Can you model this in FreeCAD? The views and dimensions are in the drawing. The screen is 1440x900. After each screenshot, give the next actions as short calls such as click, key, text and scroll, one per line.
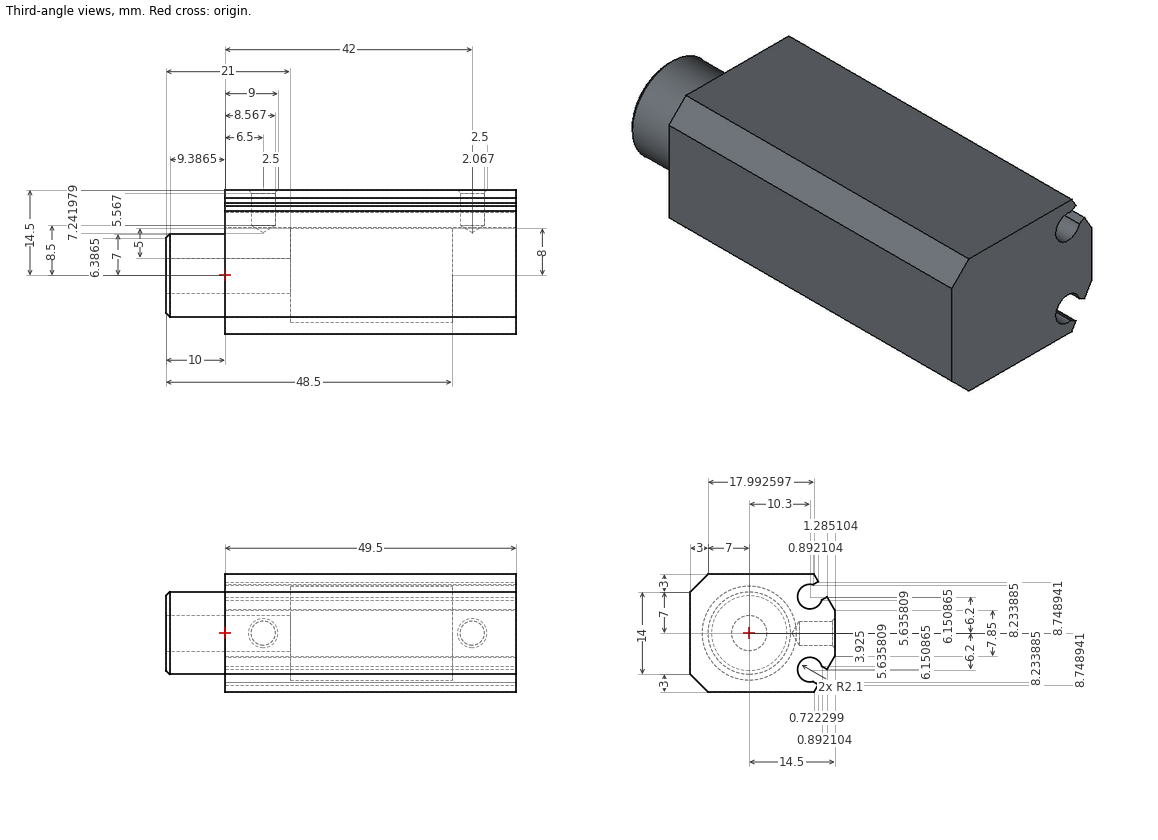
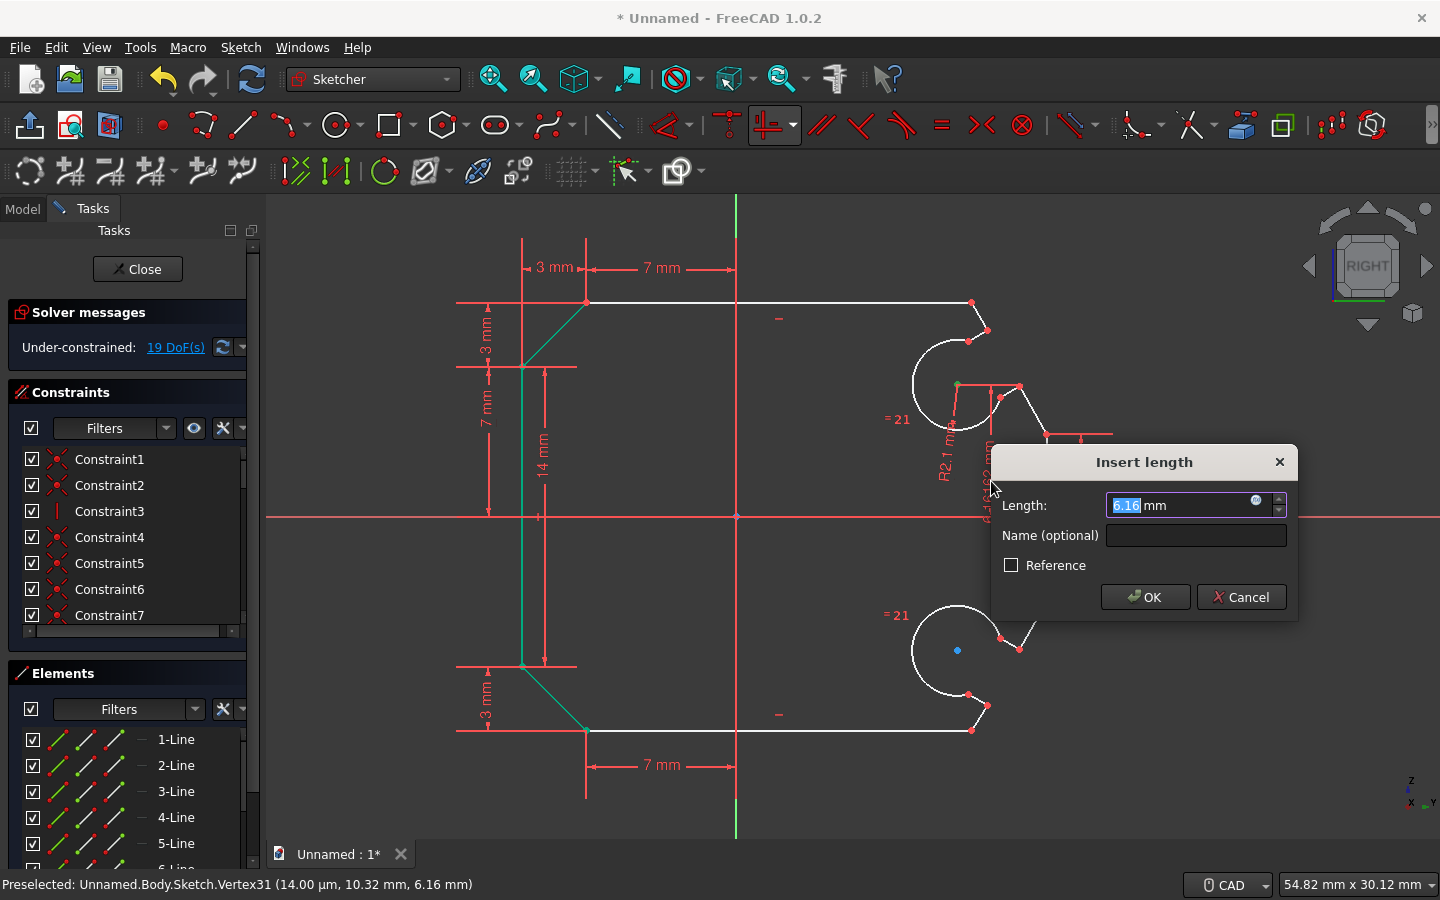
text(6.2)
key(Return)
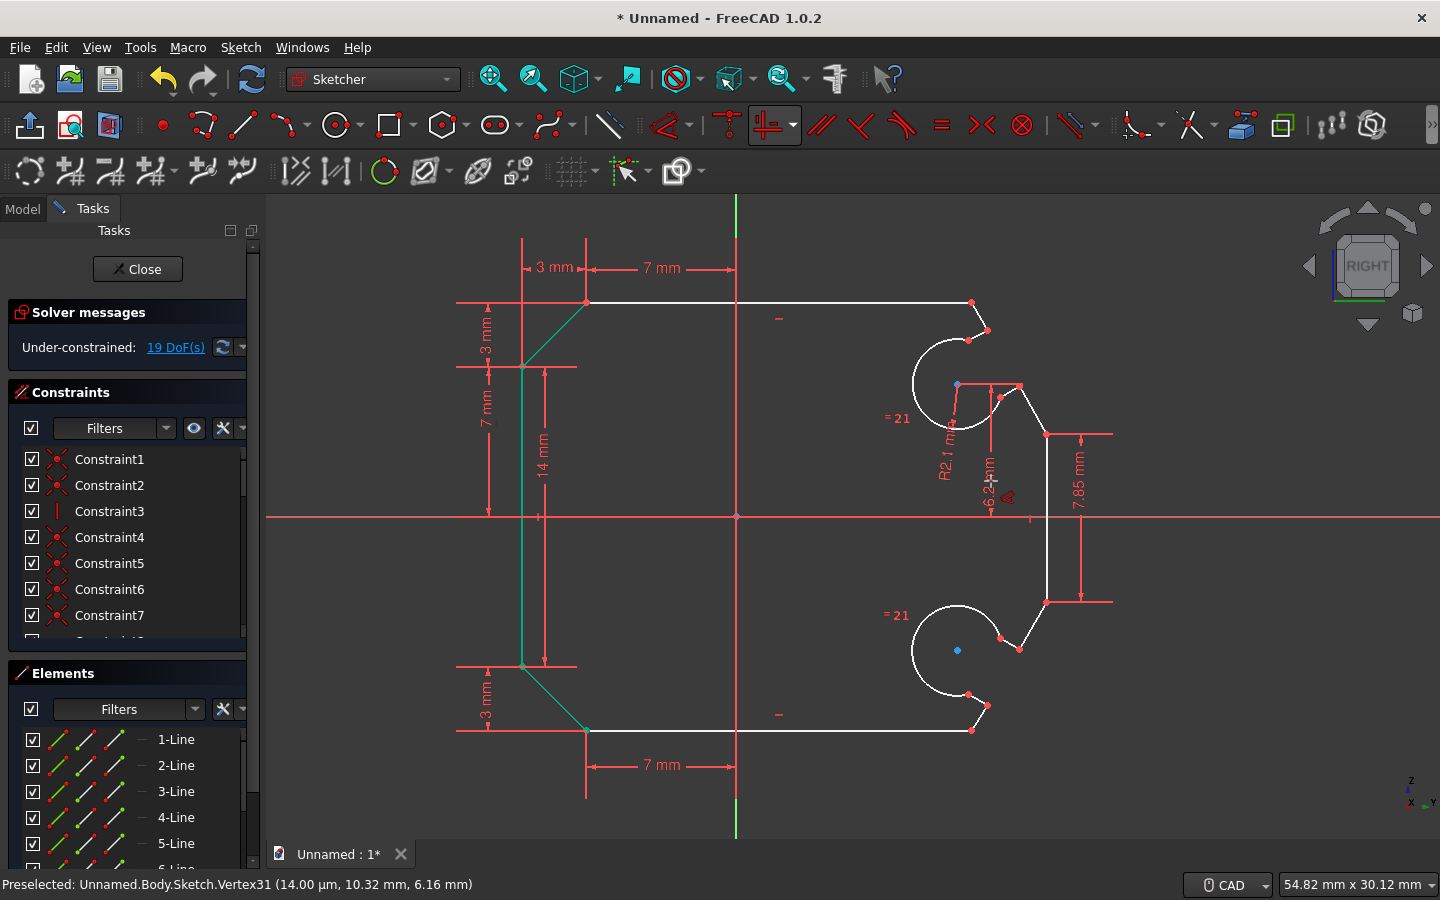
click(957, 651)
click(991, 584)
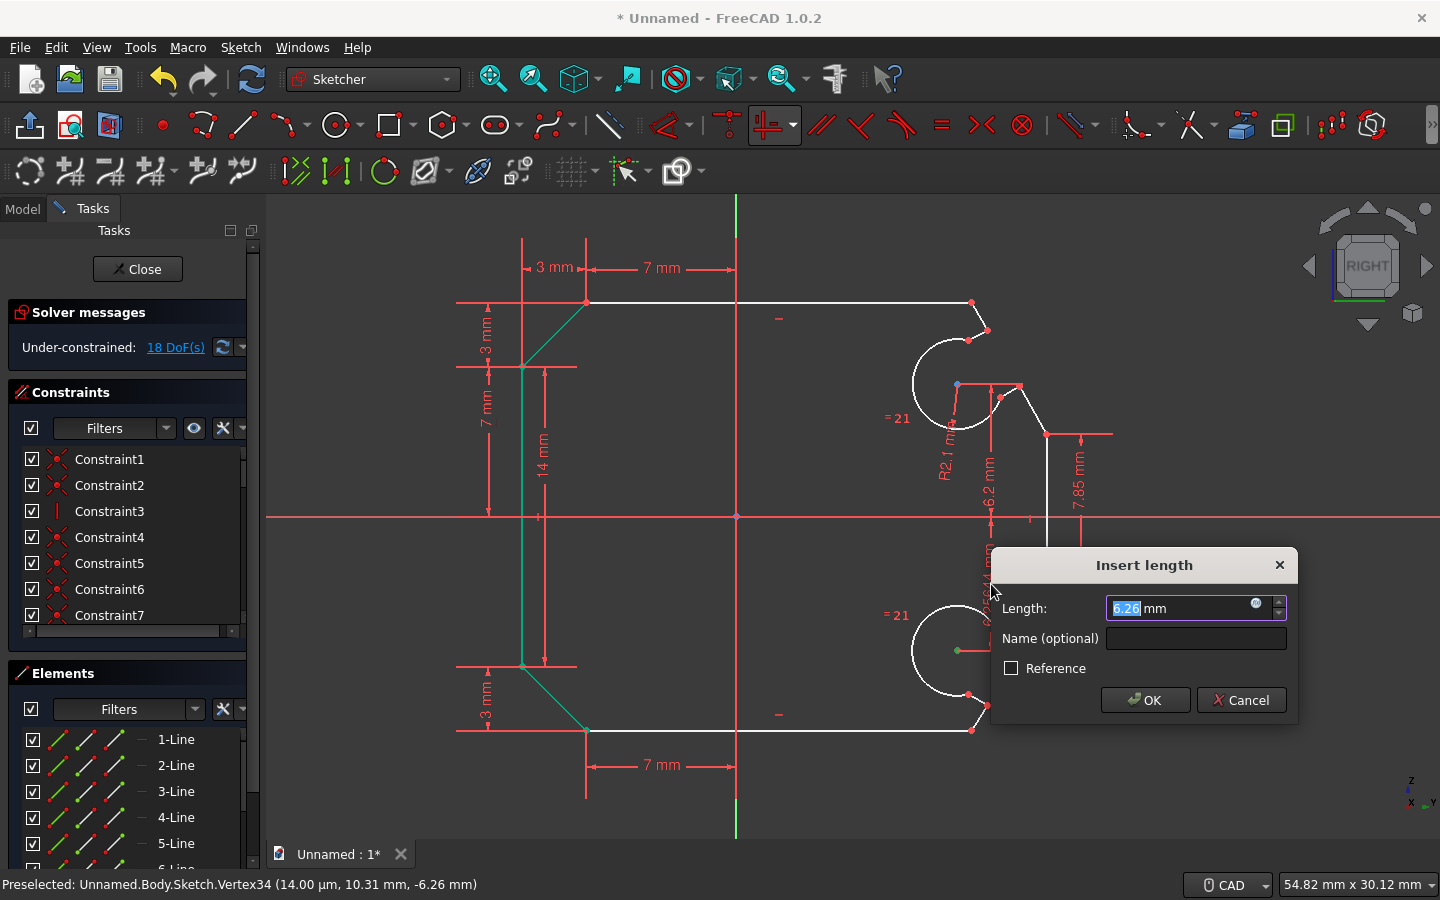
text(6.2)
key(Return)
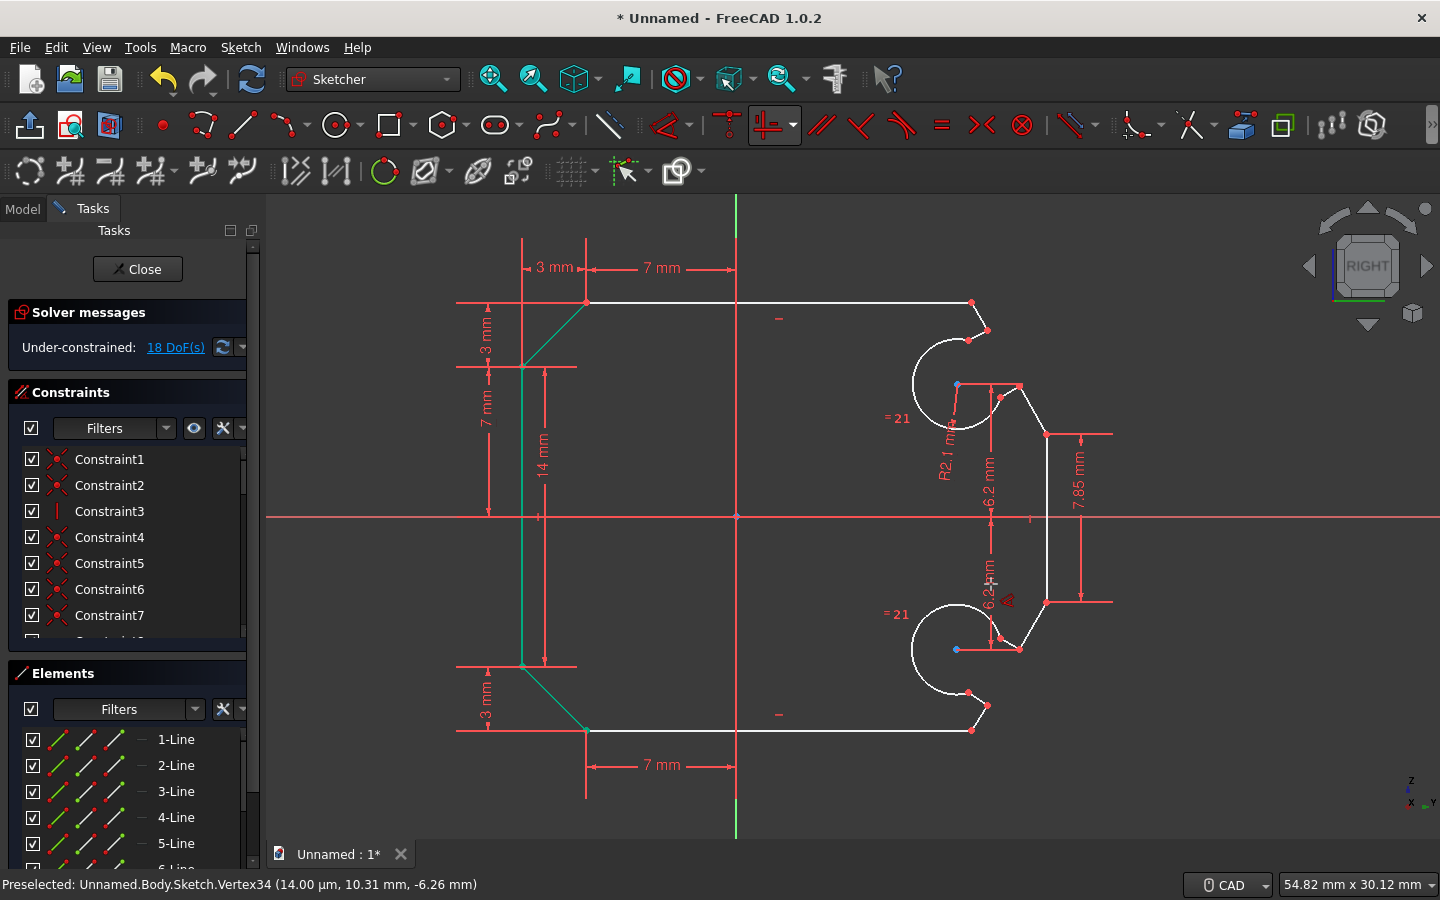
click(1047, 602)
click(892, 636)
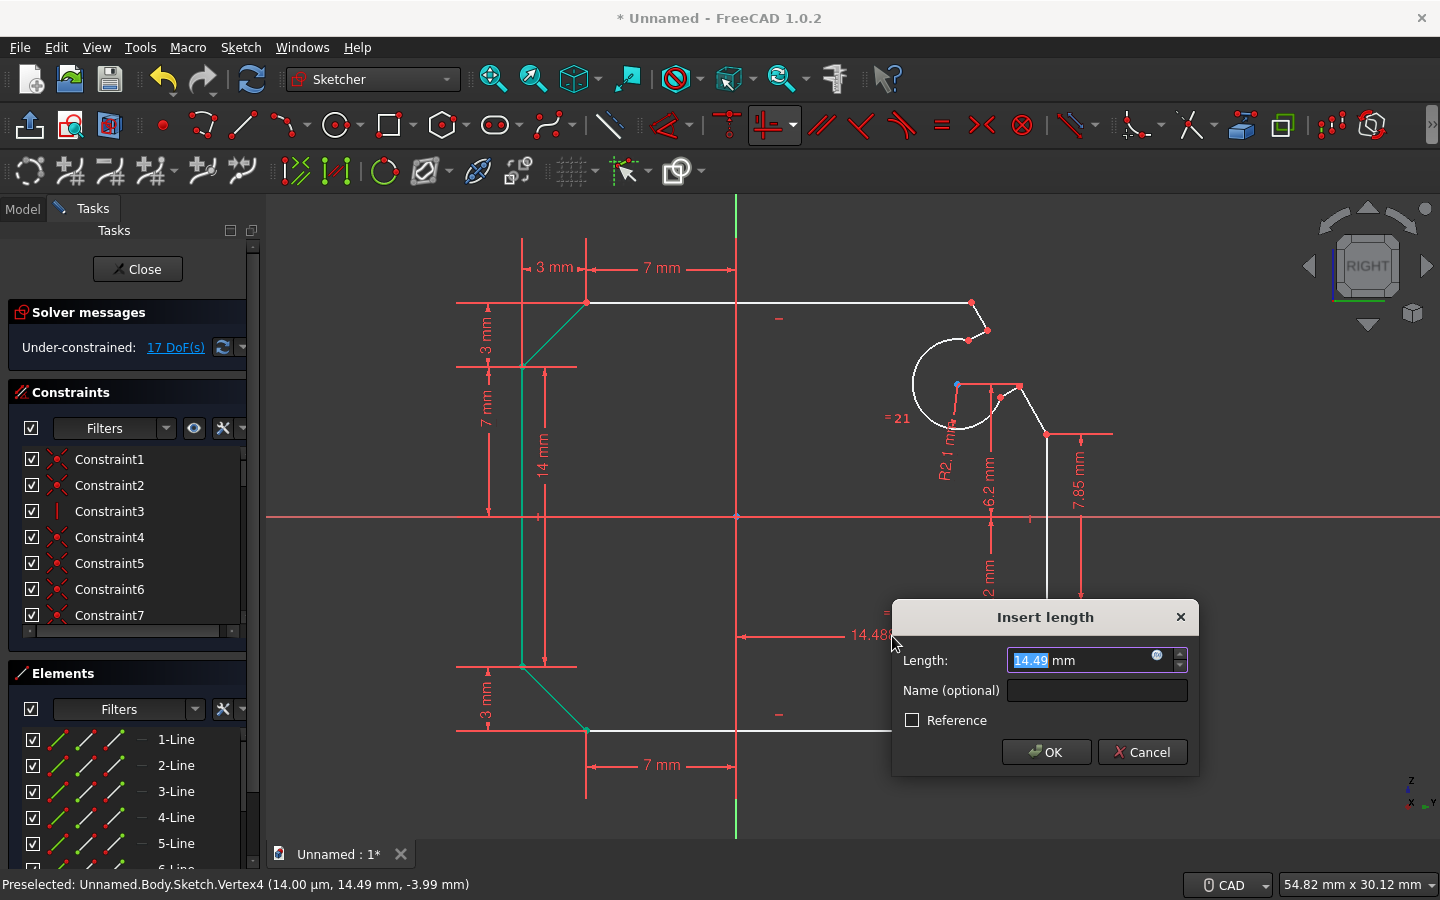
text(14.5)
key(Return)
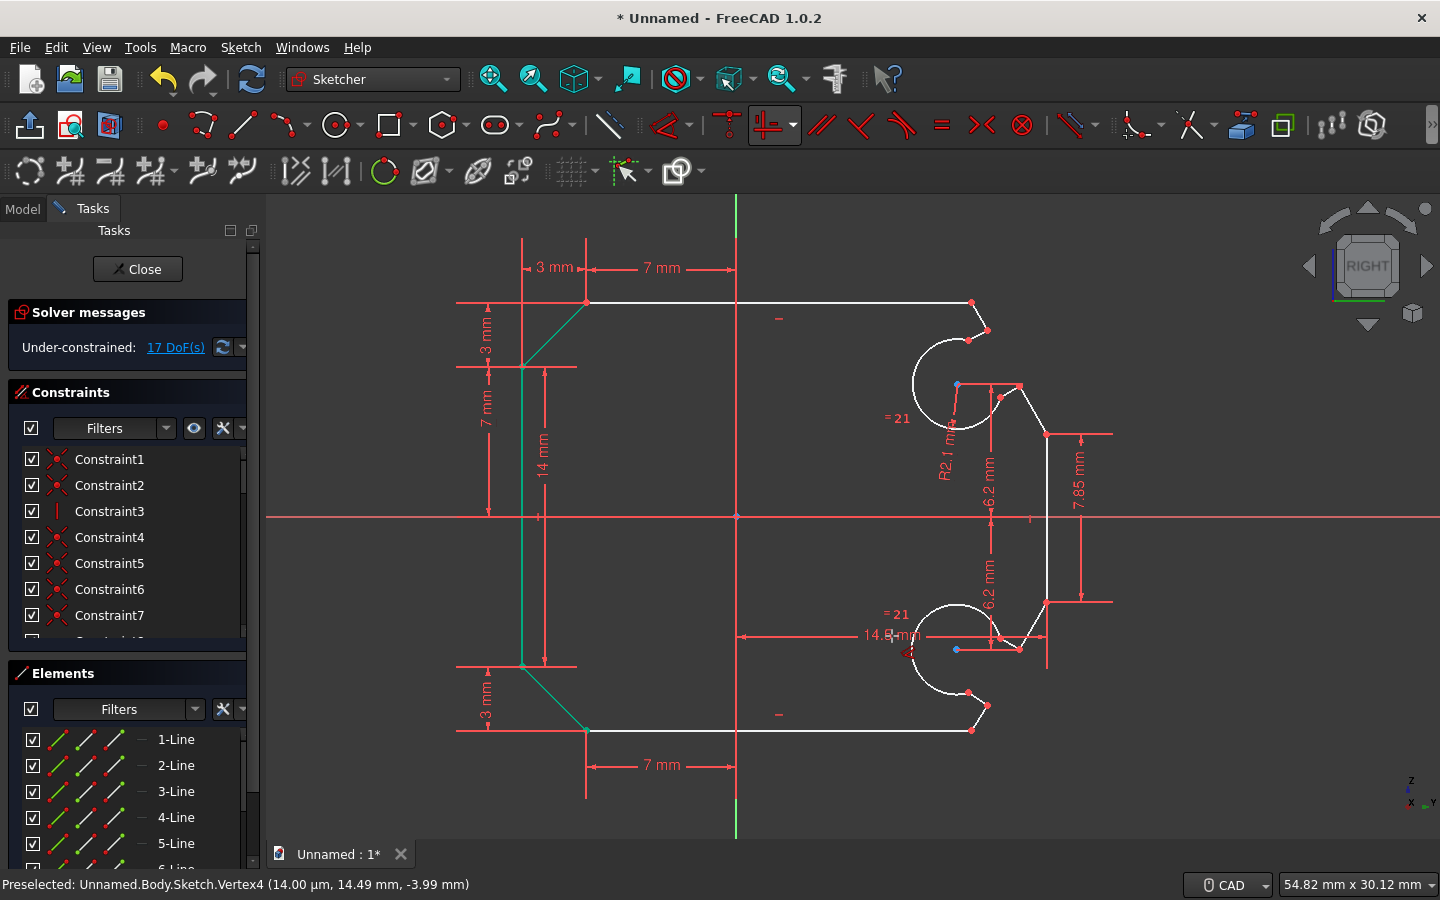
click(958, 384)
click(847, 350)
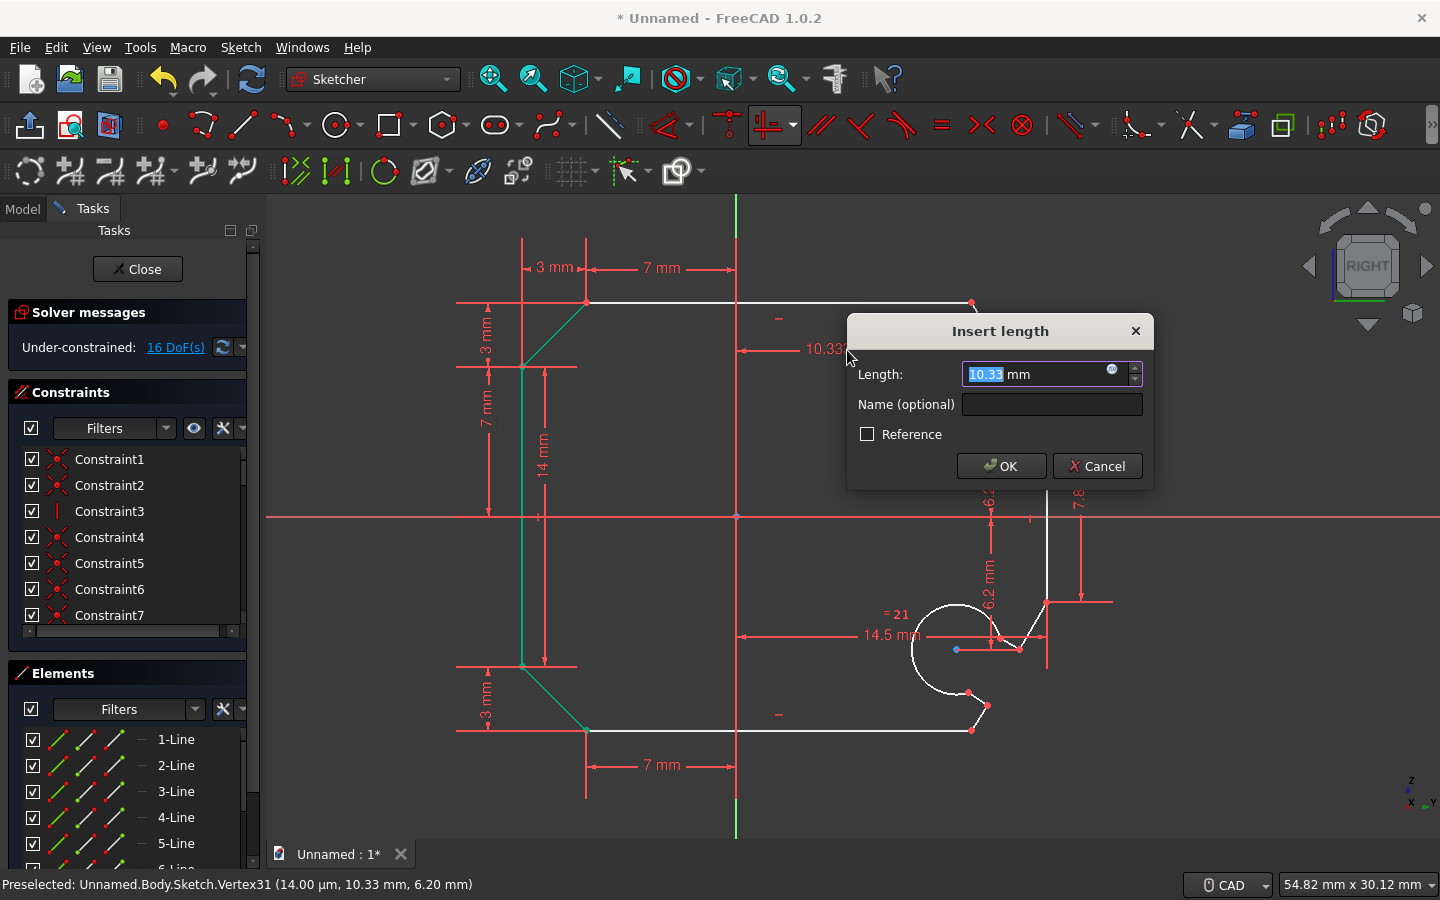
text(10.3)
key(Return)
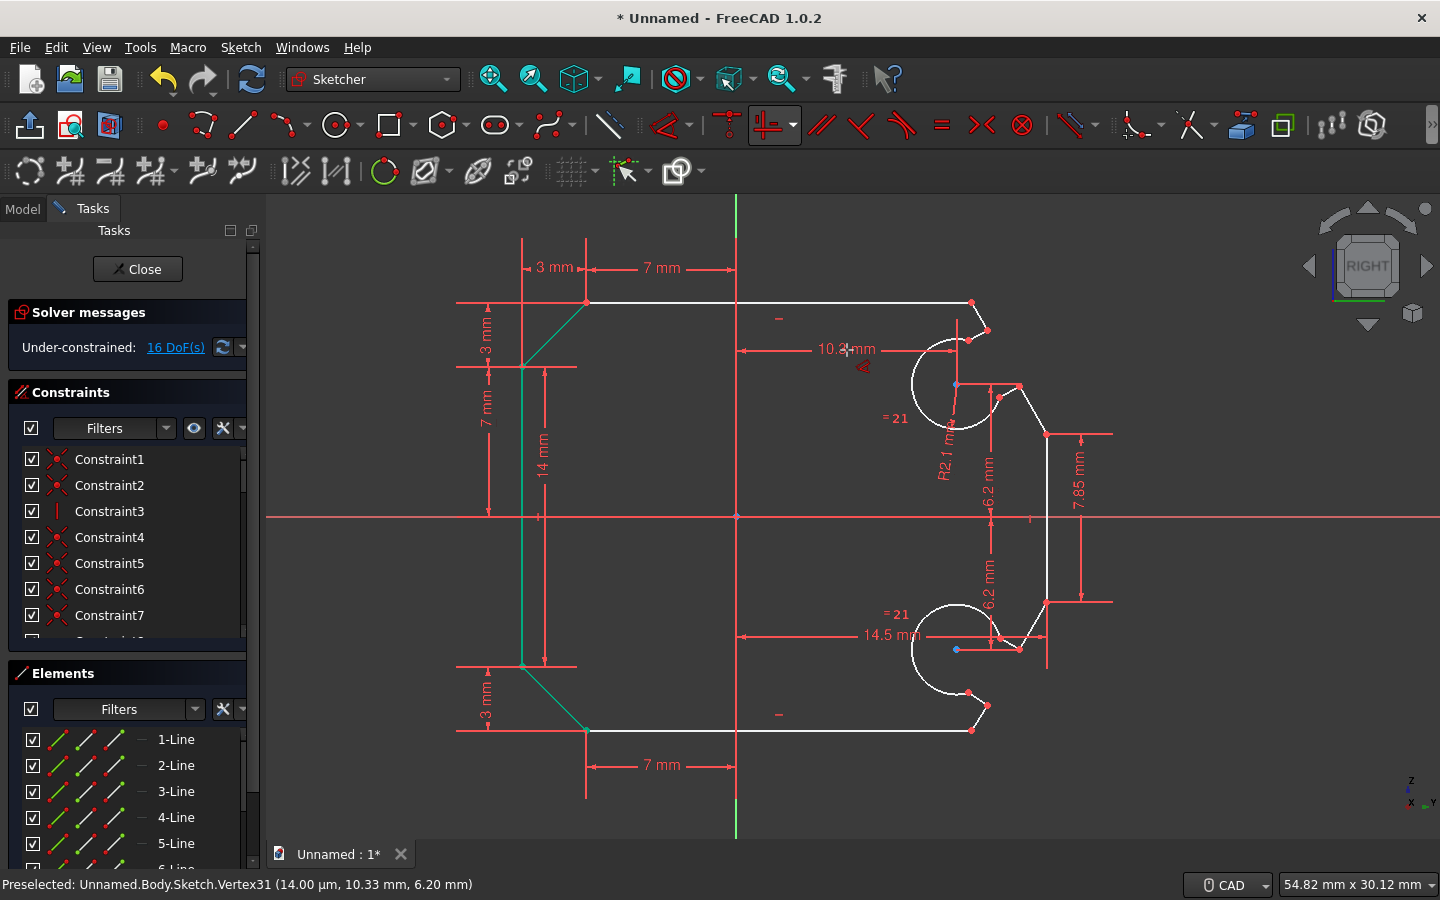
click(957, 650)
click(847, 684)